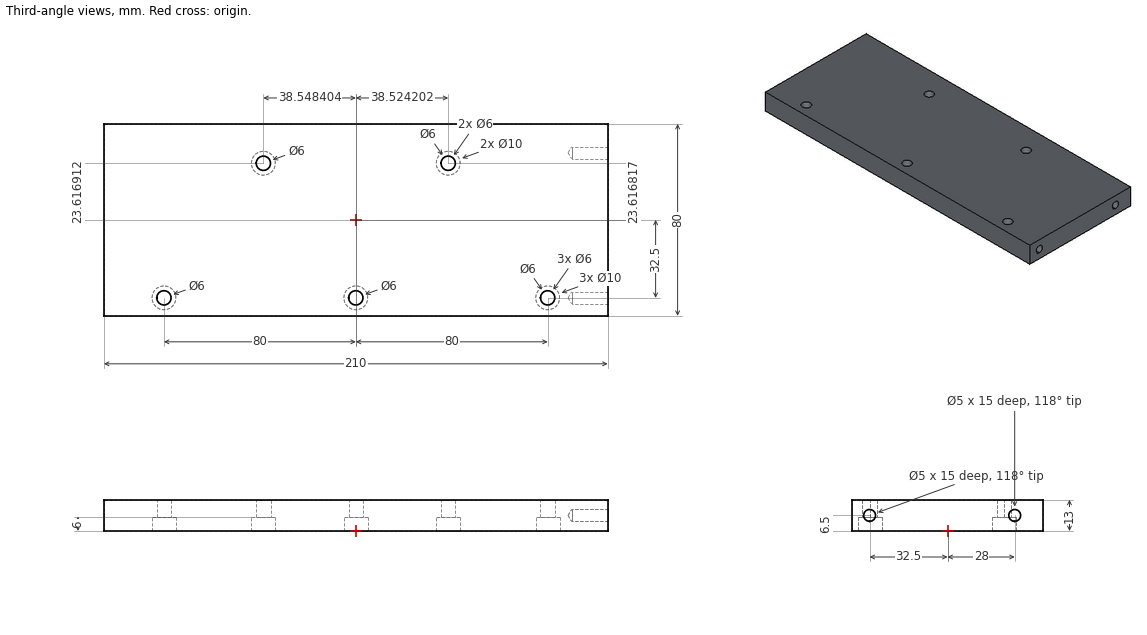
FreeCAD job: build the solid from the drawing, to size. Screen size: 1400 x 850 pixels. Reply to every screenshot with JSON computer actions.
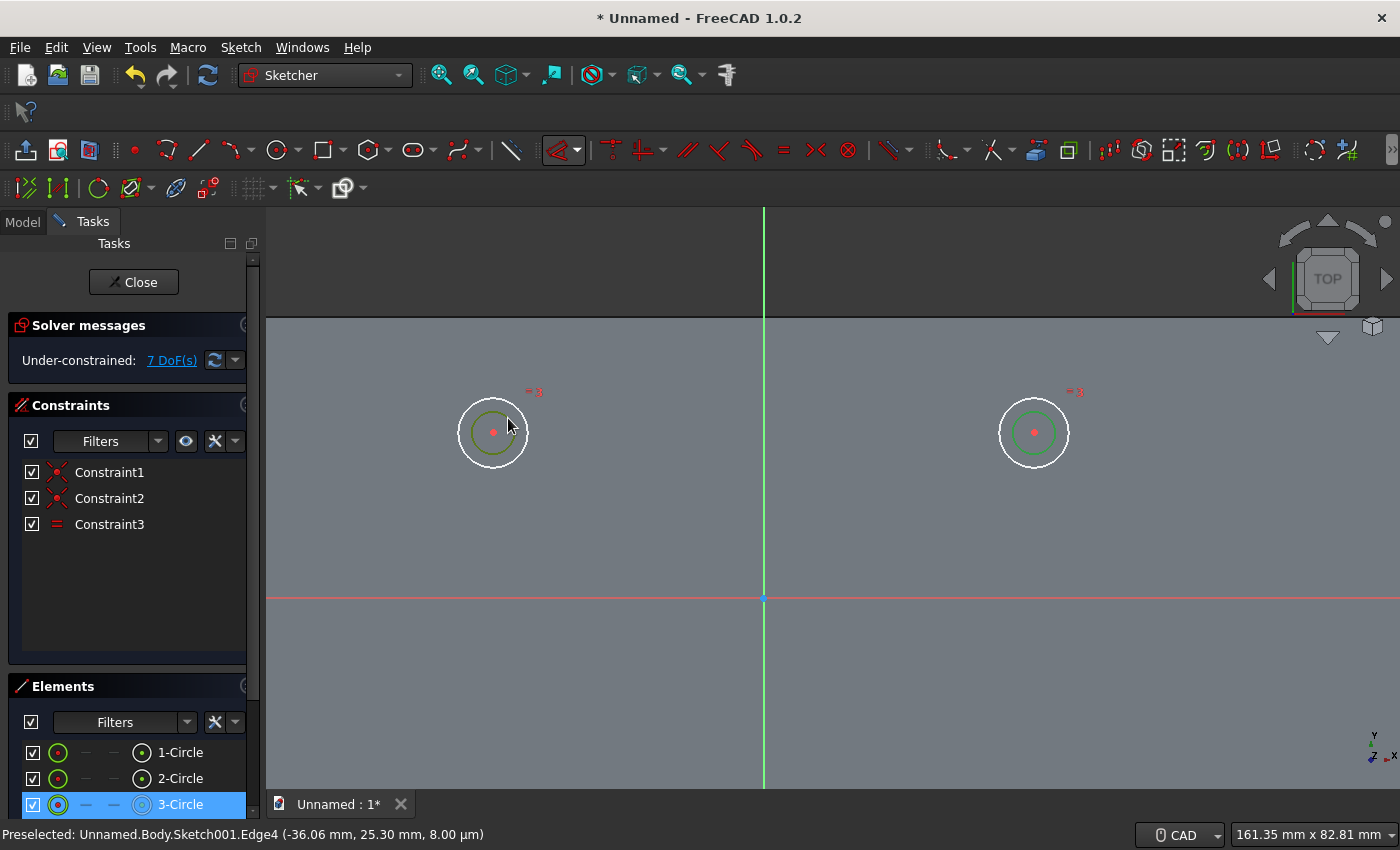
{"action": "key", "text": "e"}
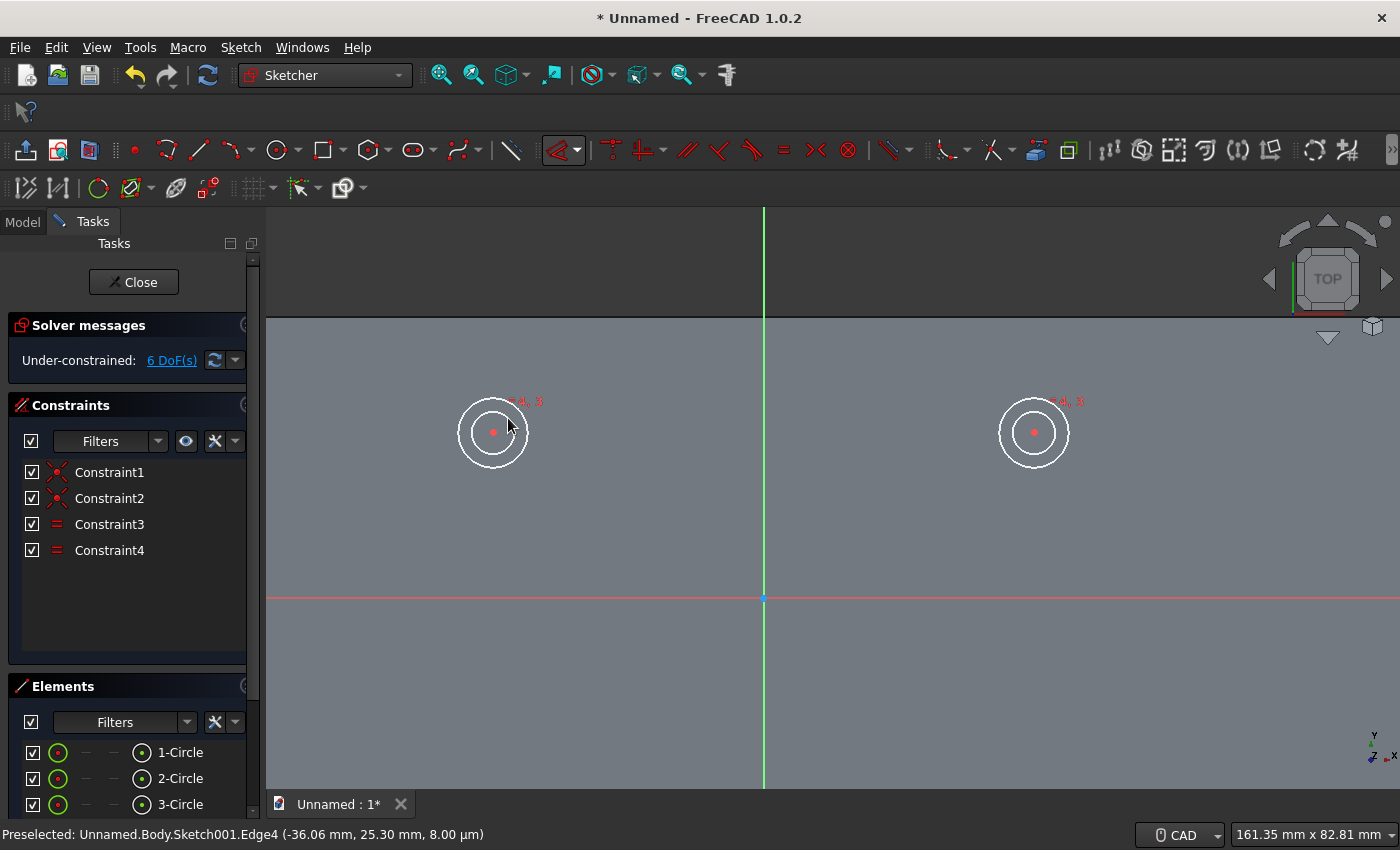
{"action": "key", "text": "d"}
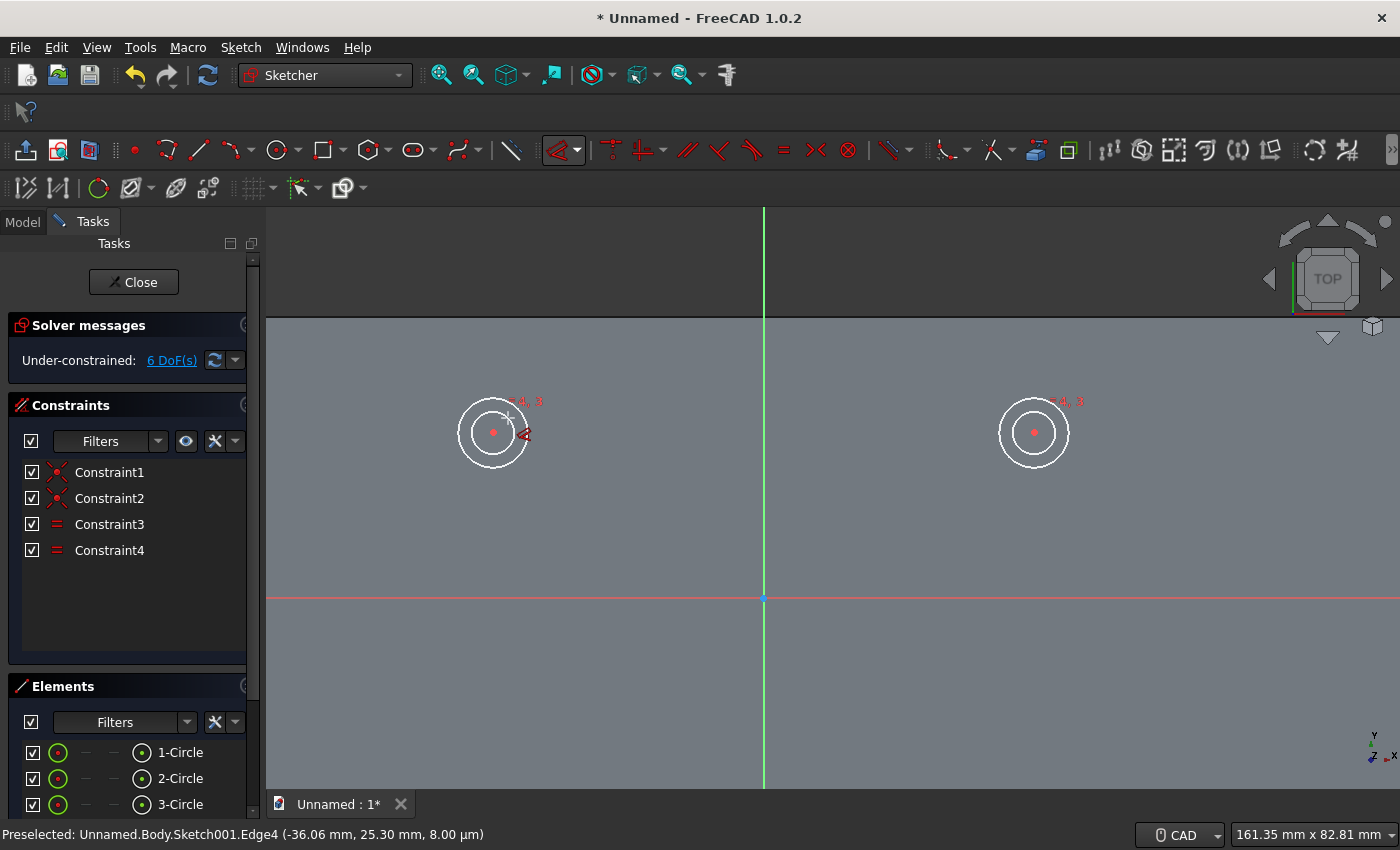
{"action": "left_click", "coordinate": [1058, 408]}
{"action": "left_click", "coordinate": [1080, 385]}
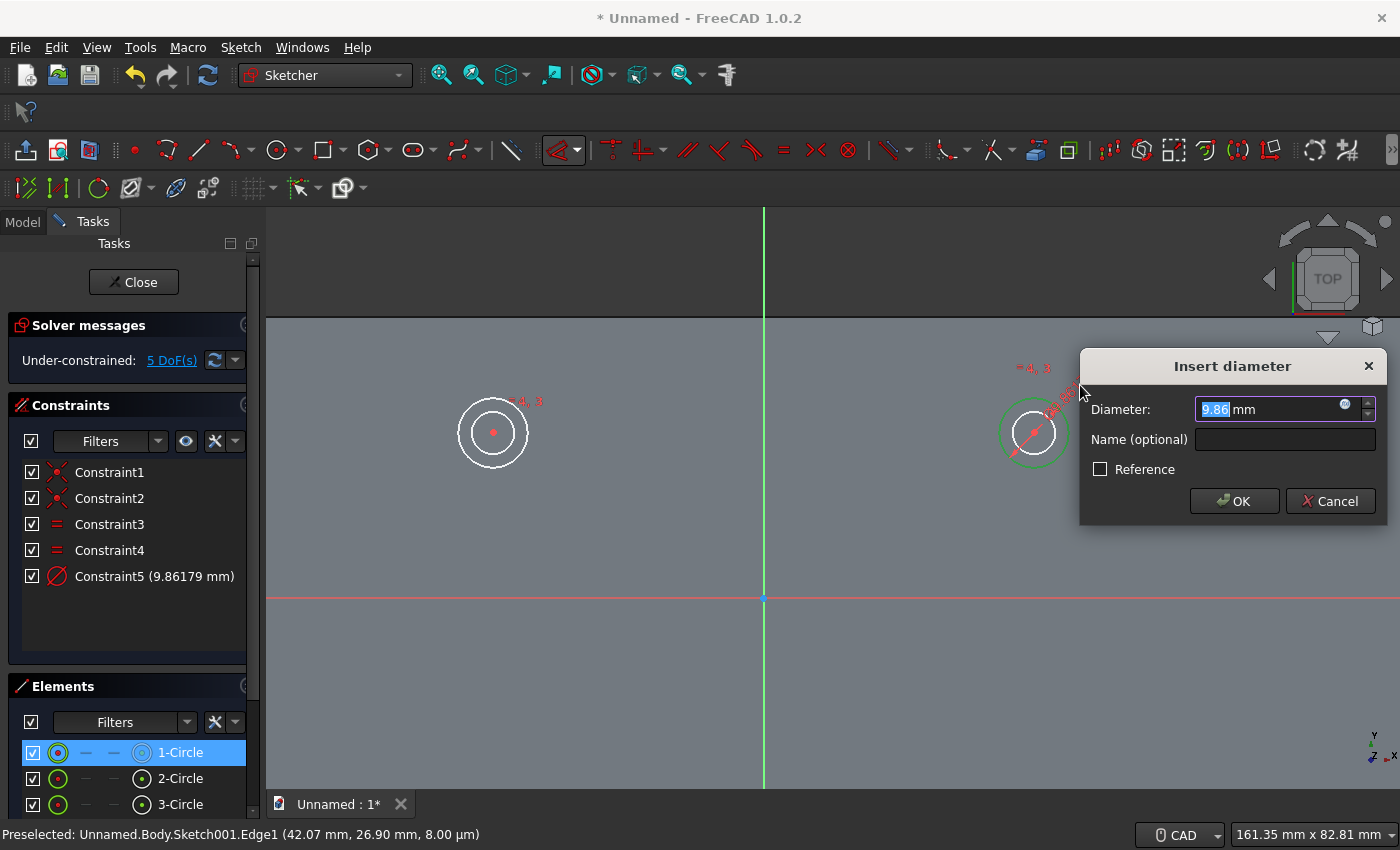
{"action": "type", "text": "10"}
{"action": "key", "text": "Return"}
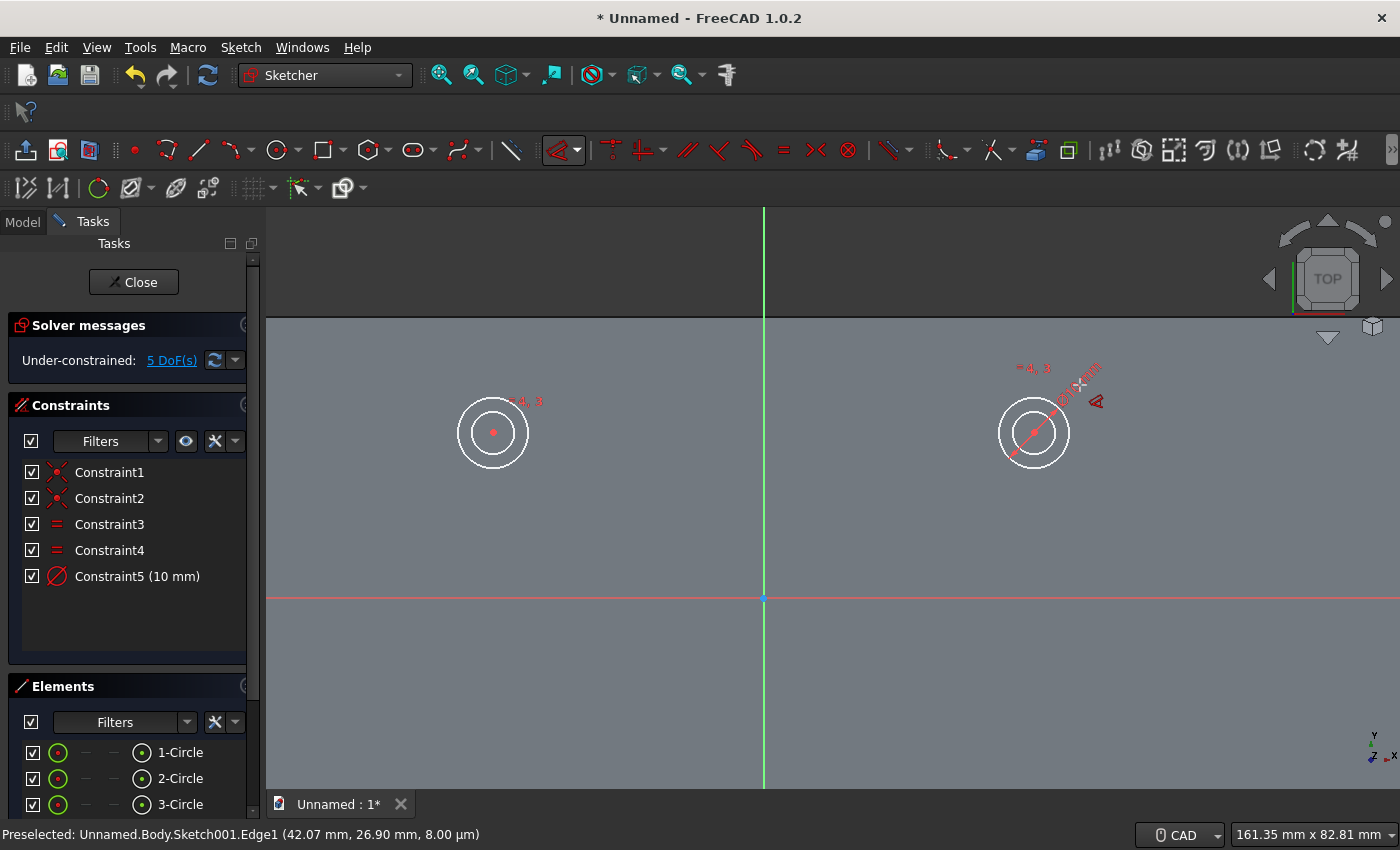
{"action": "left_click", "coordinate": [1049, 418]}
{"action": "left_click", "coordinate": [1085, 418]}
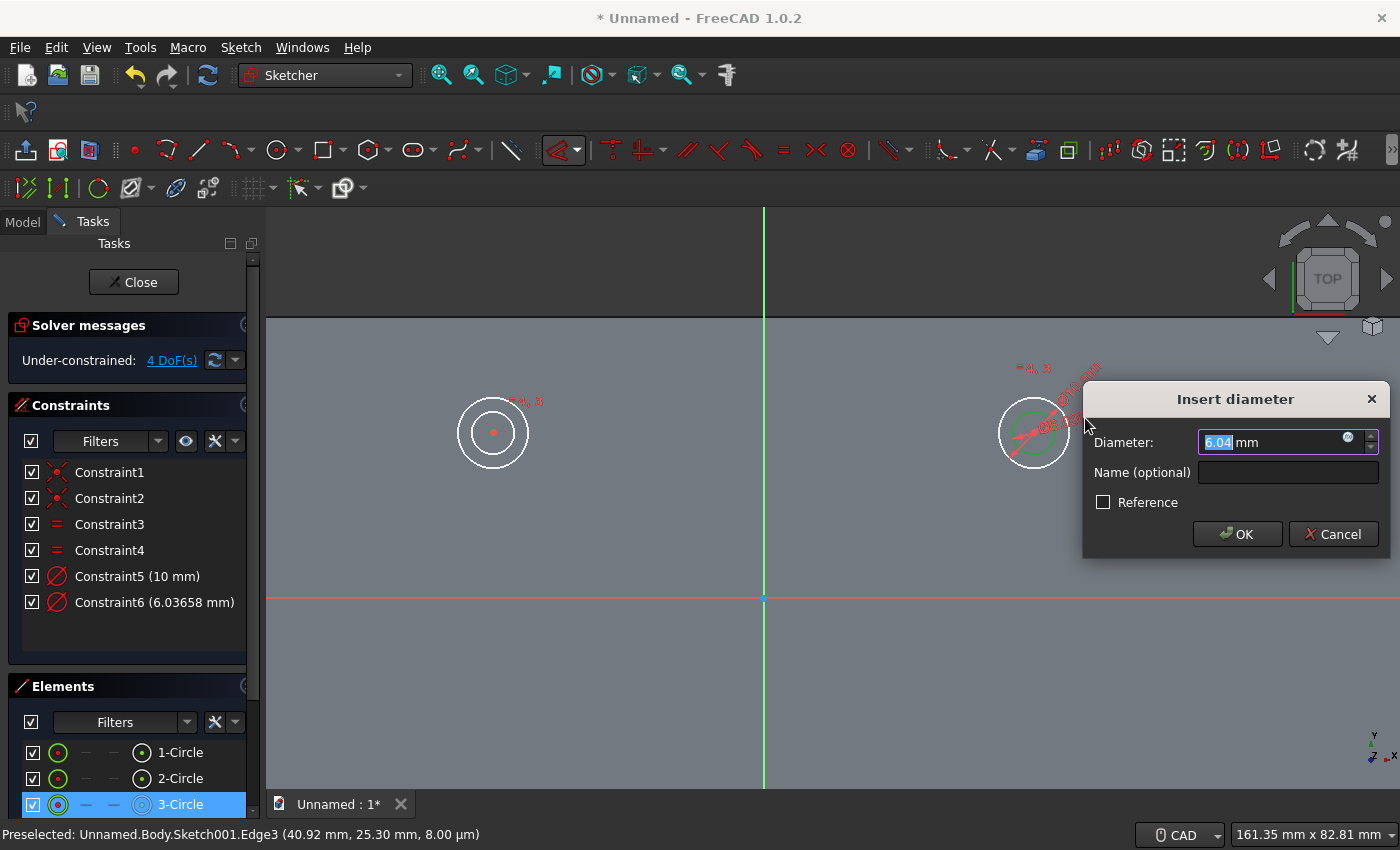
{"action": "type", "text": "6"}
{"action": "key", "text": "Return"}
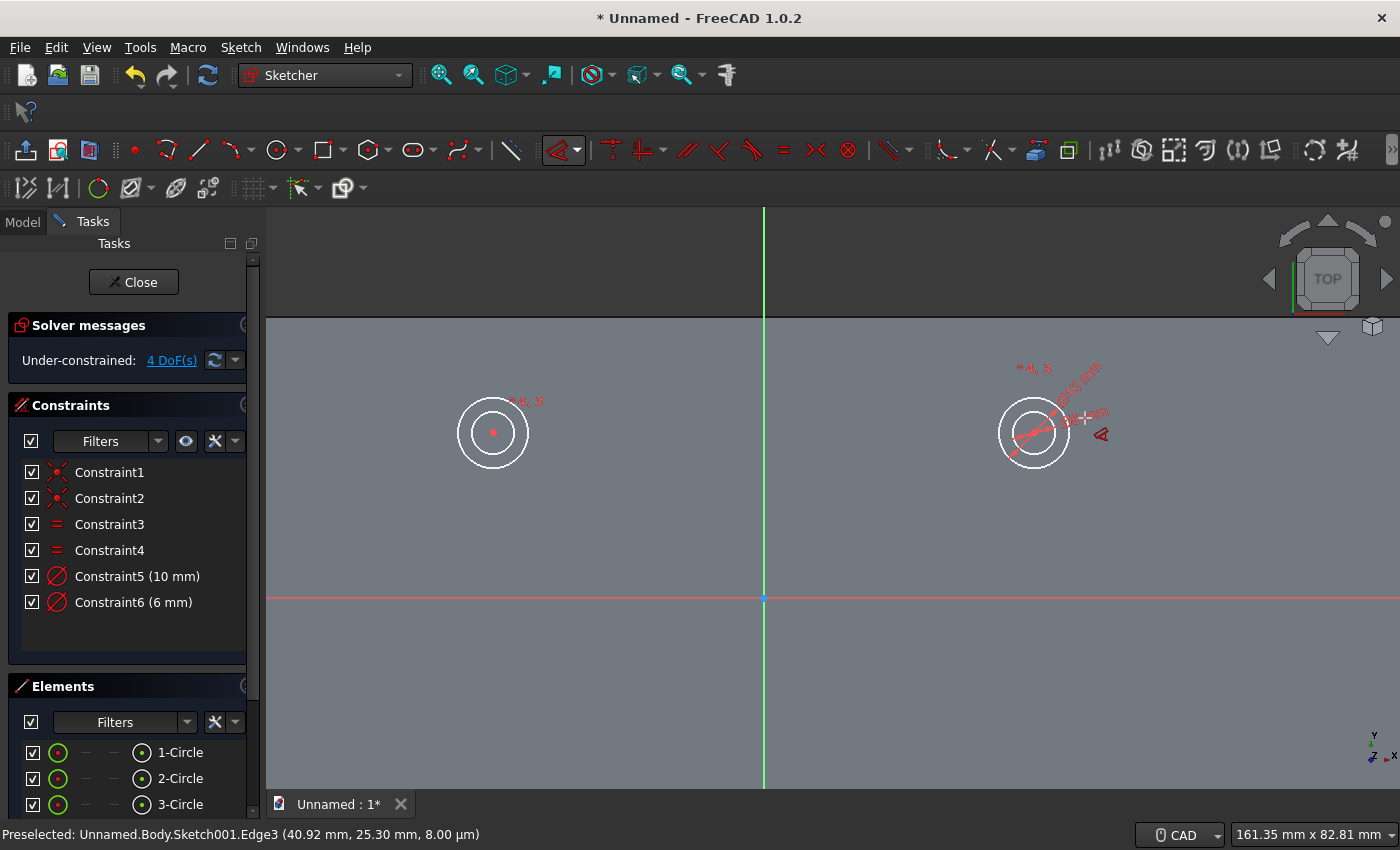
{"action": "left_click", "coordinate": [1034, 433]}
{"action": "left_click", "coordinate": [899, 632]}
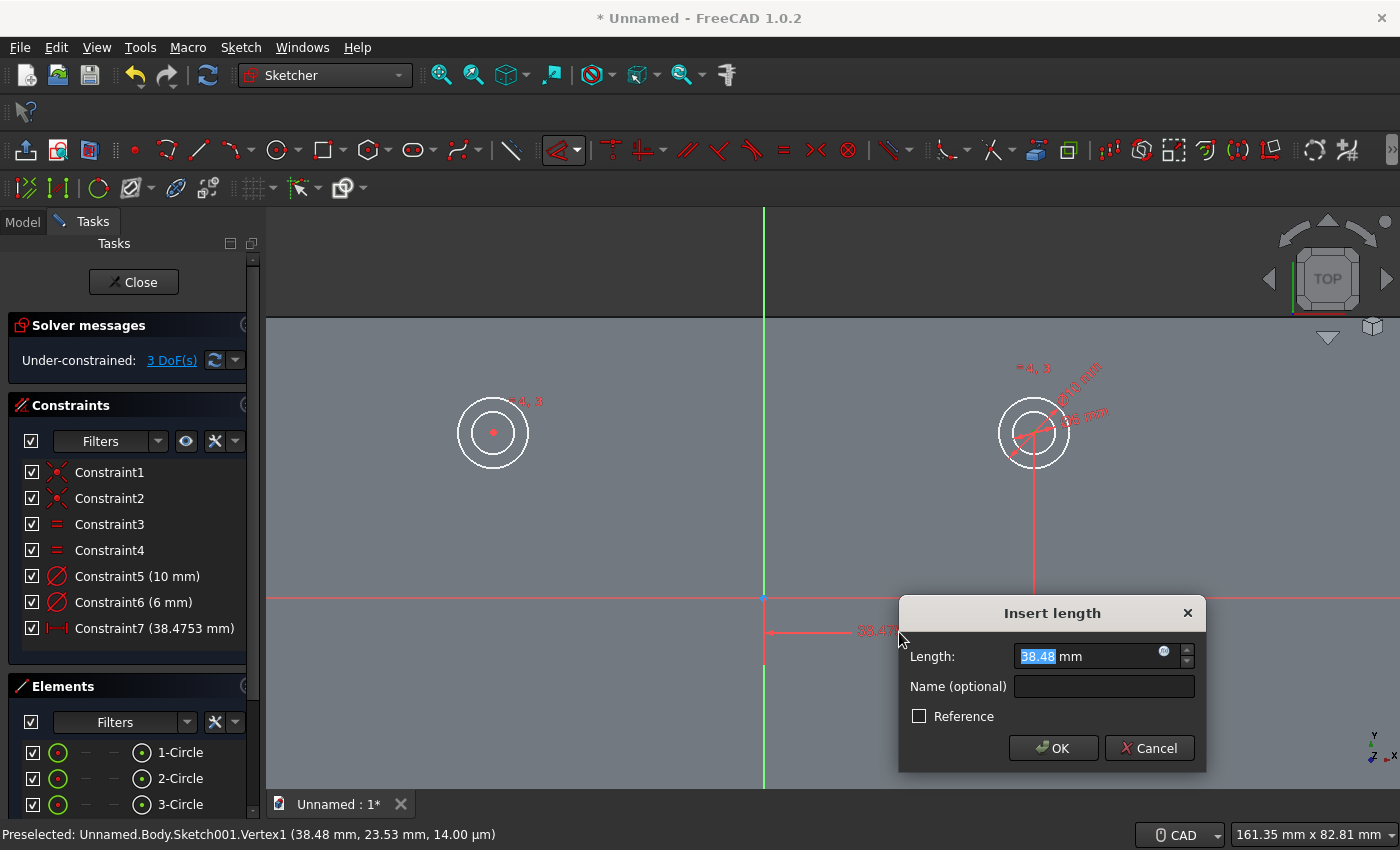
{"action": "type", "text": "38.524202"}
{"action": "key", "text": "Return"}